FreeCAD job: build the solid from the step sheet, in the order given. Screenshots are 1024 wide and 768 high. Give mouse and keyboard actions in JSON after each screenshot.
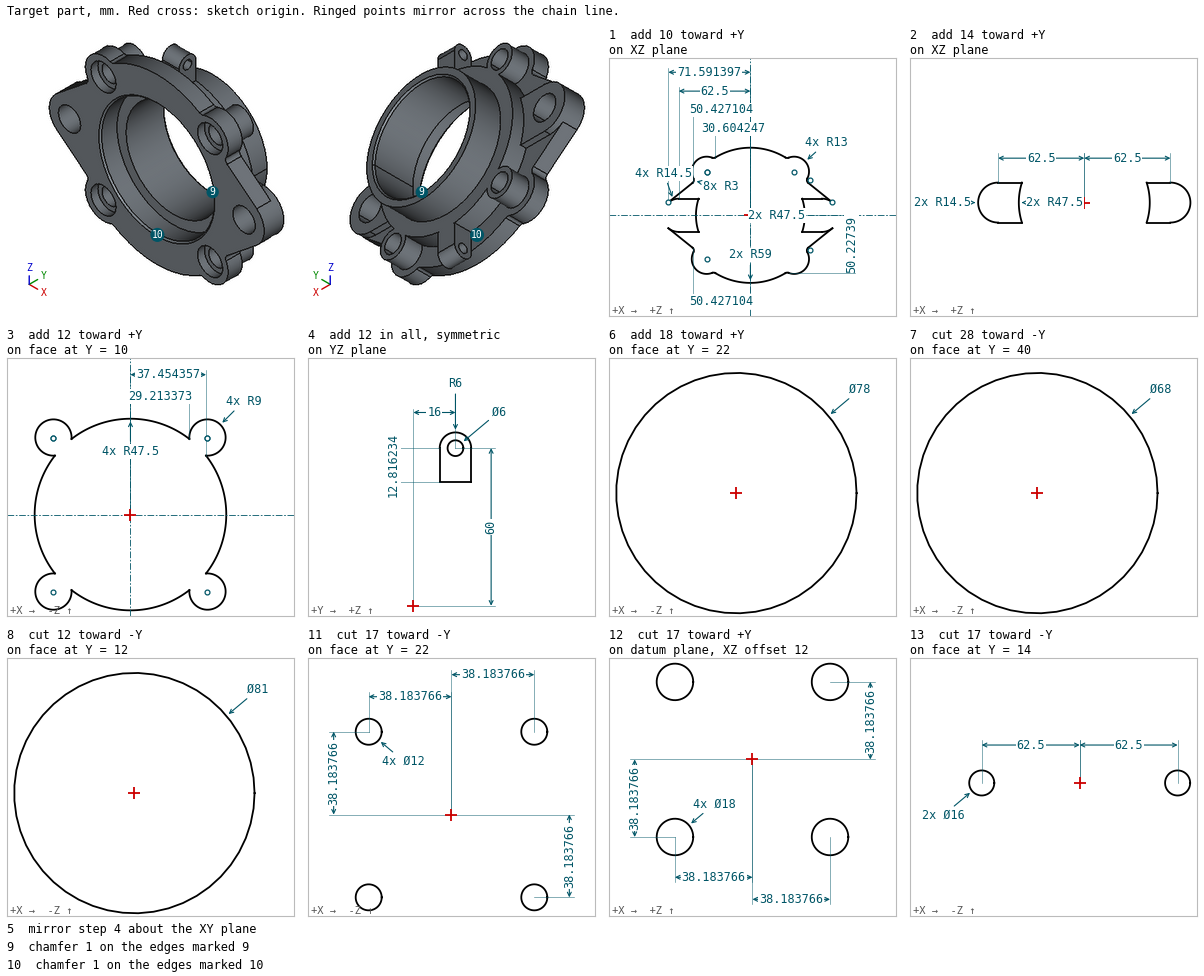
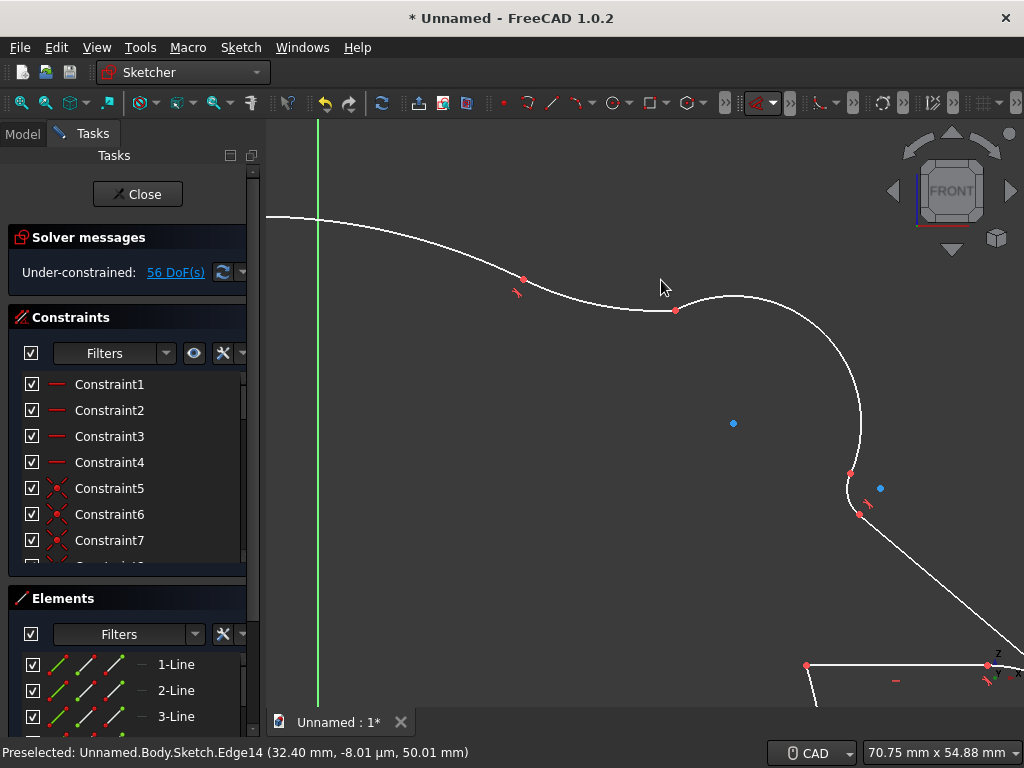
{"action": "scroll", "coordinate": [661, 281], "scroll_direction": "down", "scroll_amount": 7}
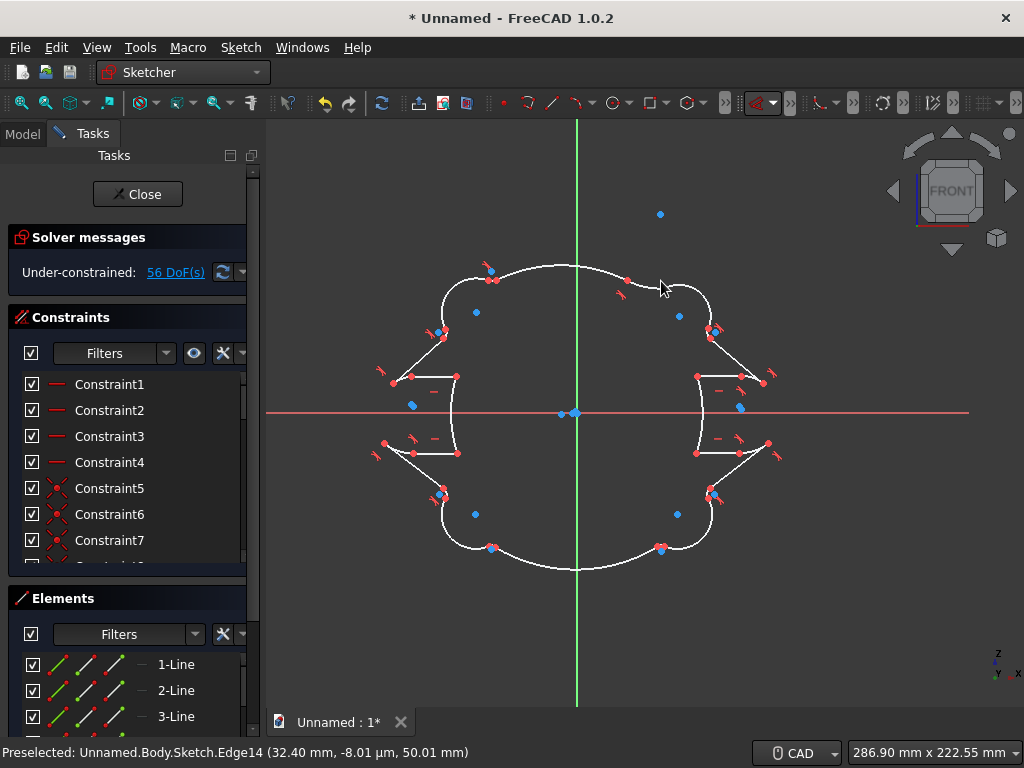
{"action": "left_click", "coordinate": [638, 285]}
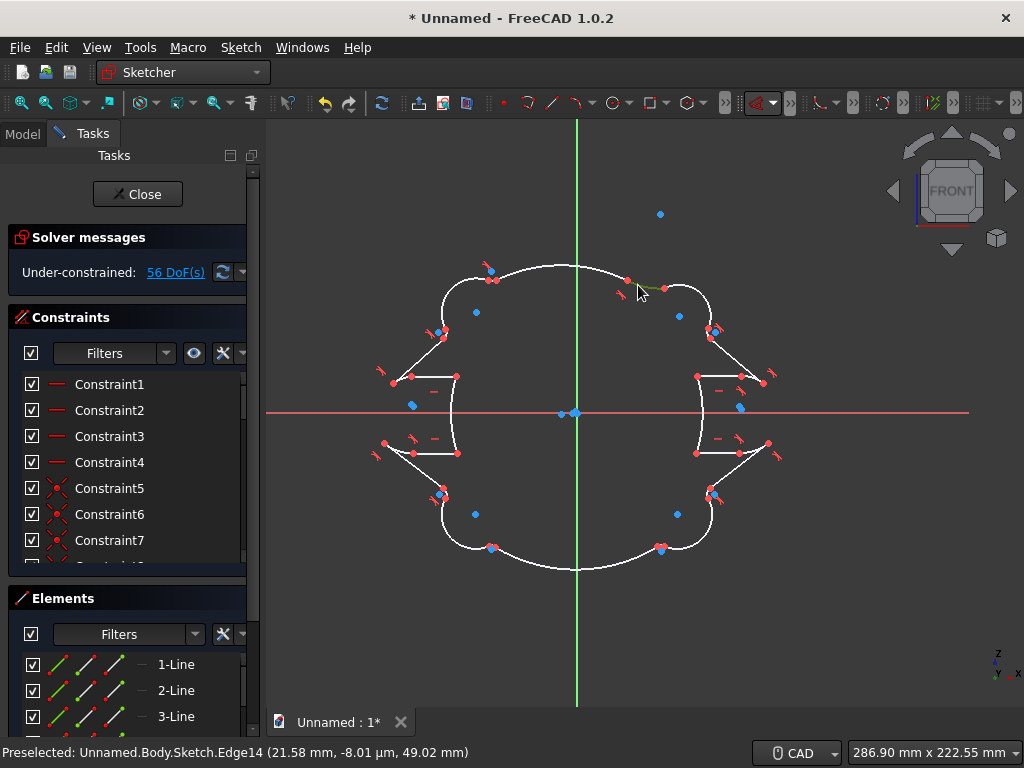
{"action": "left_click", "coordinate": [709, 306]}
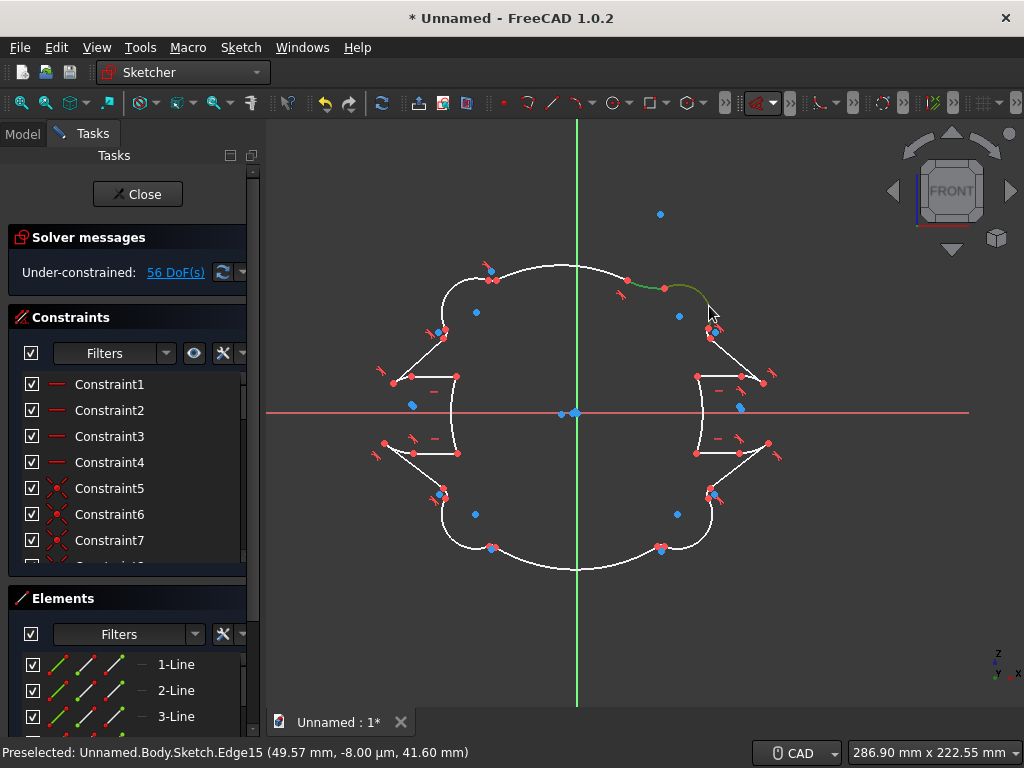
{"action": "key", "text": "t"}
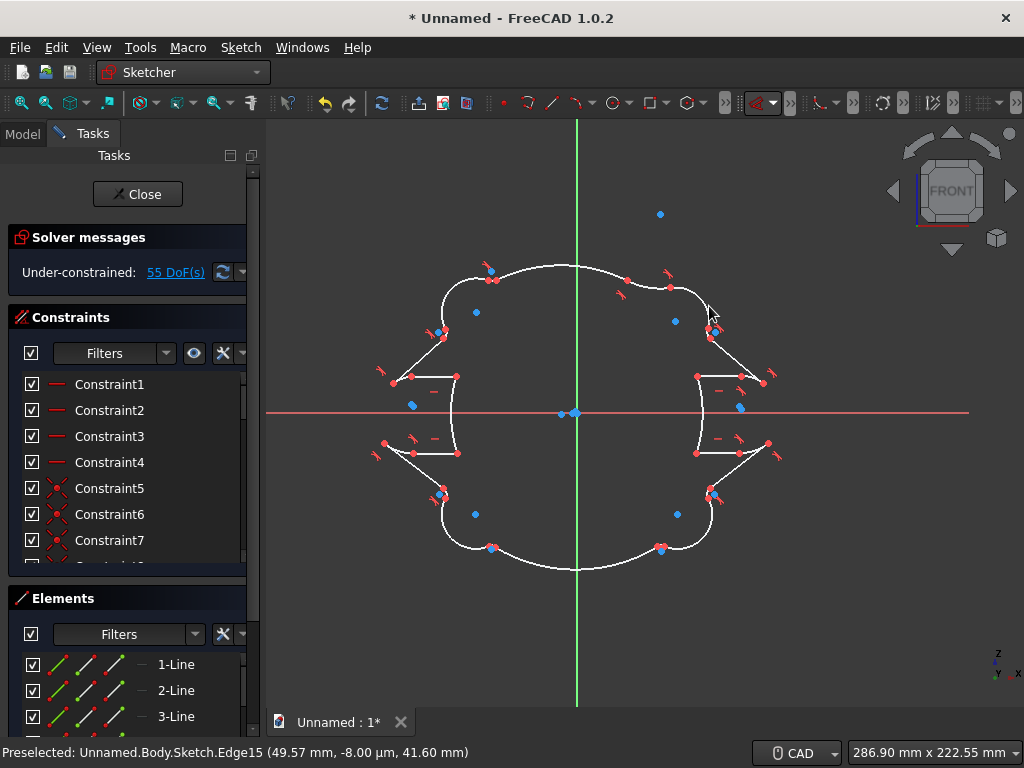
{"action": "left_click", "coordinate": [707, 309]}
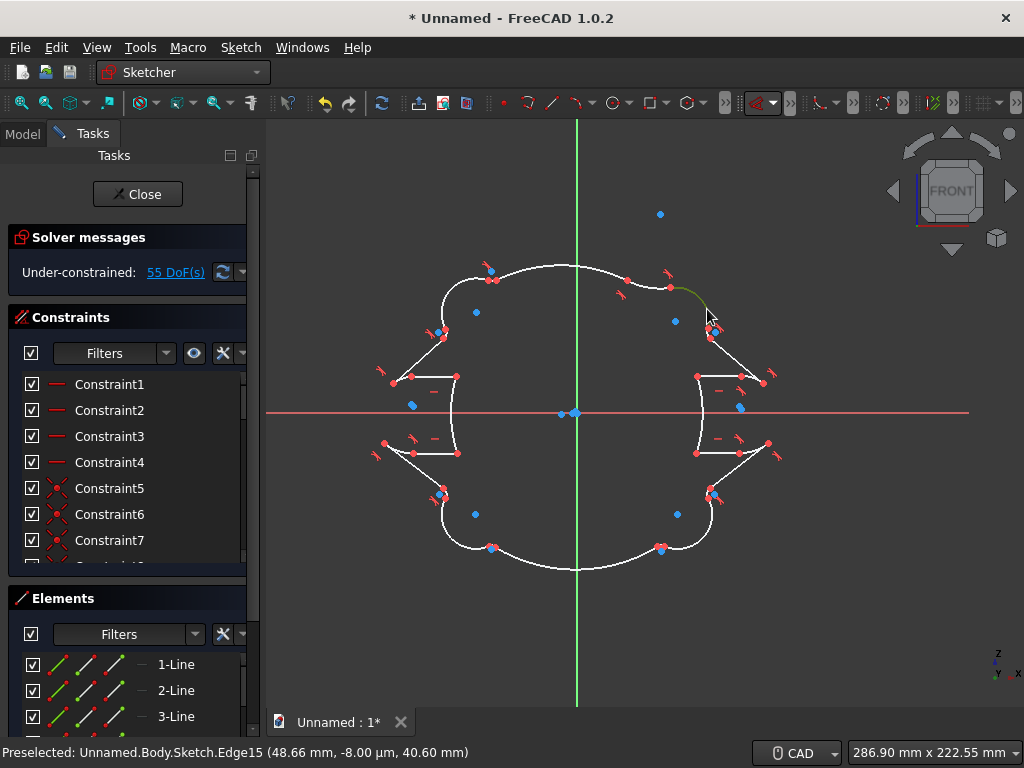
{"action": "scroll", "coordinate": [707, 334], "scroll_direction": "up", "scroll_amount": 5}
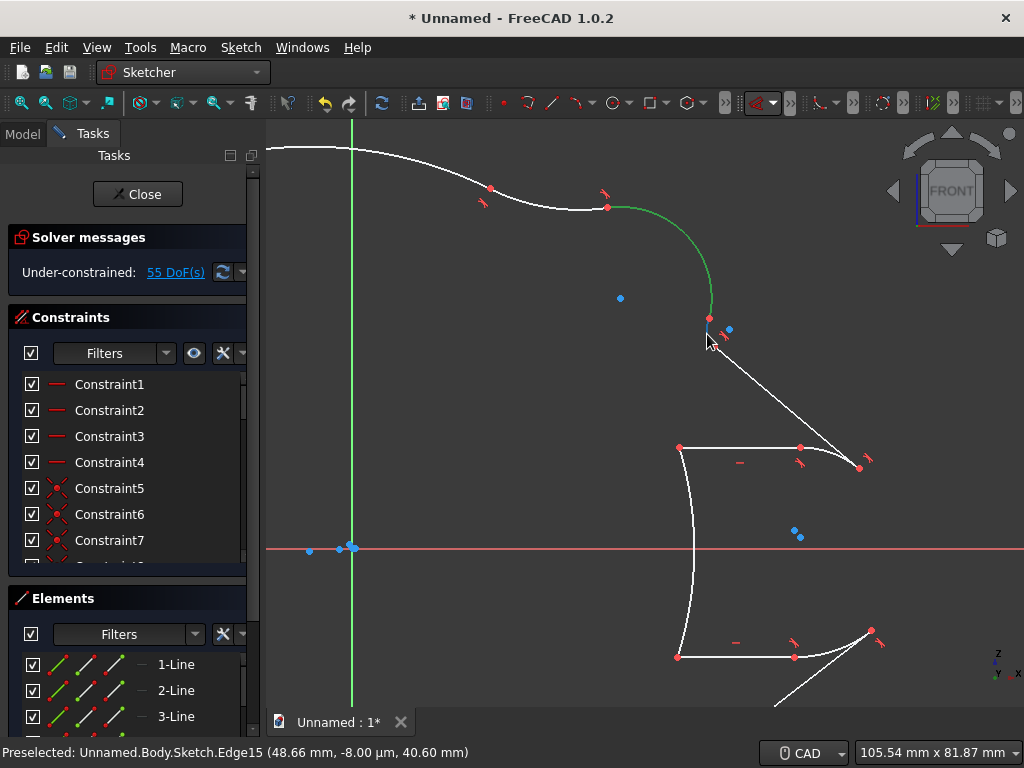
{"action": "left_click", "coordinate": [707, 334]}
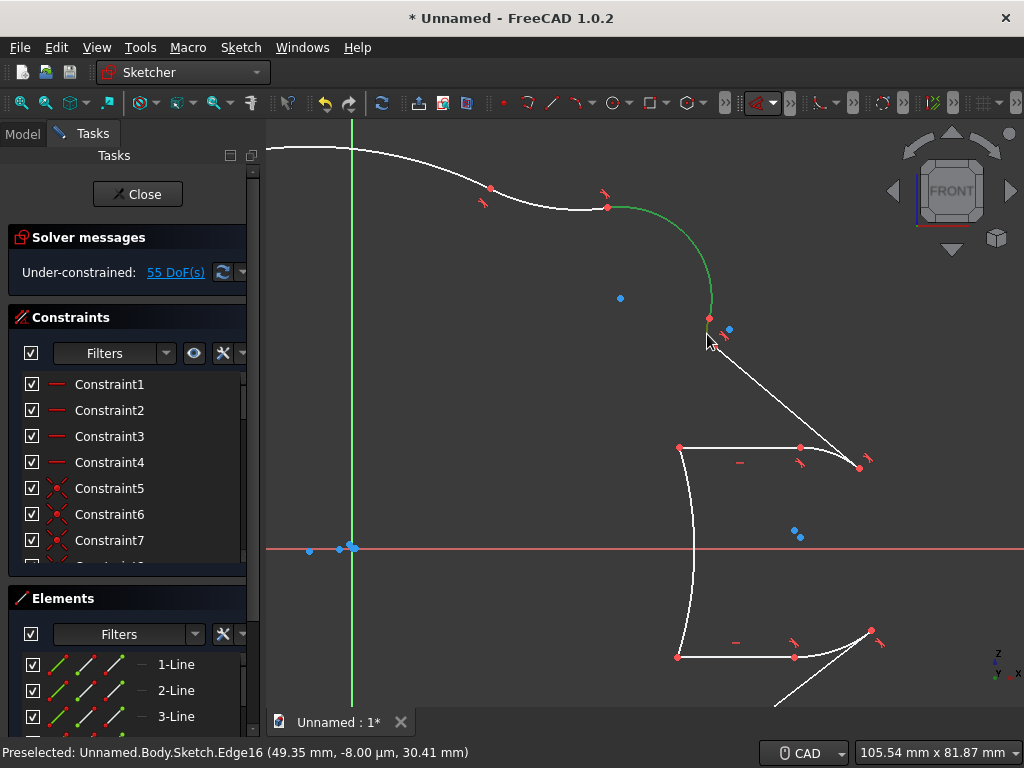
{"action": "key", "text": "t"}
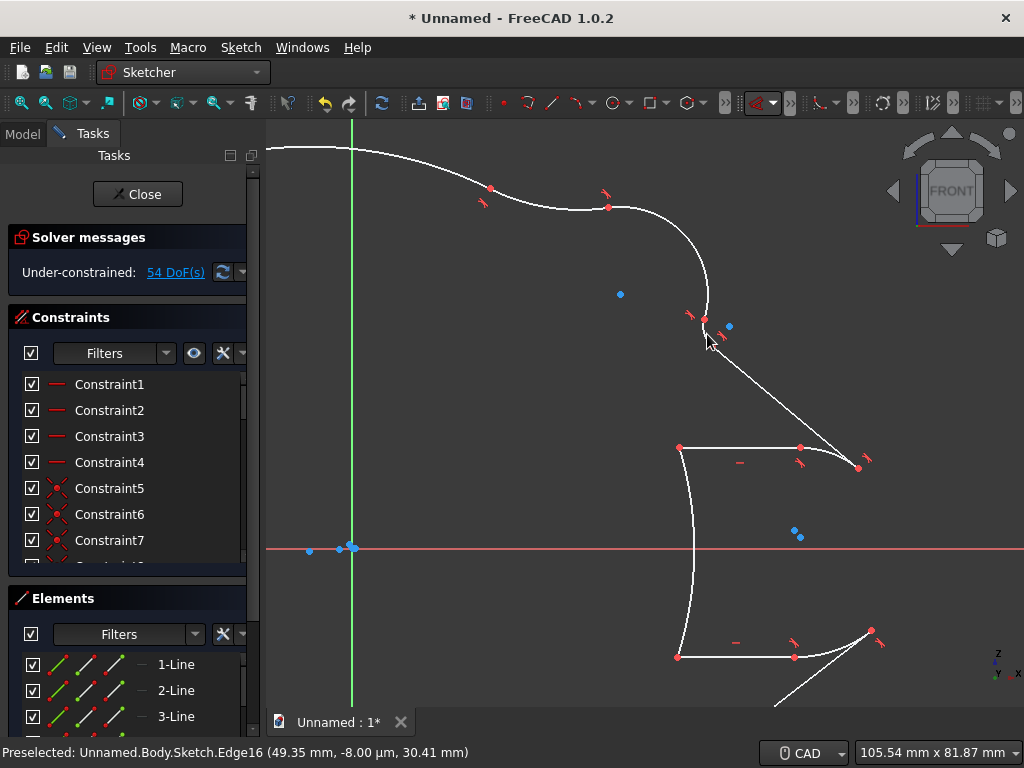
{"action": "scroll", "coordinate": [707, 334], "scroll_direction": "down", "scroll_amount": 5}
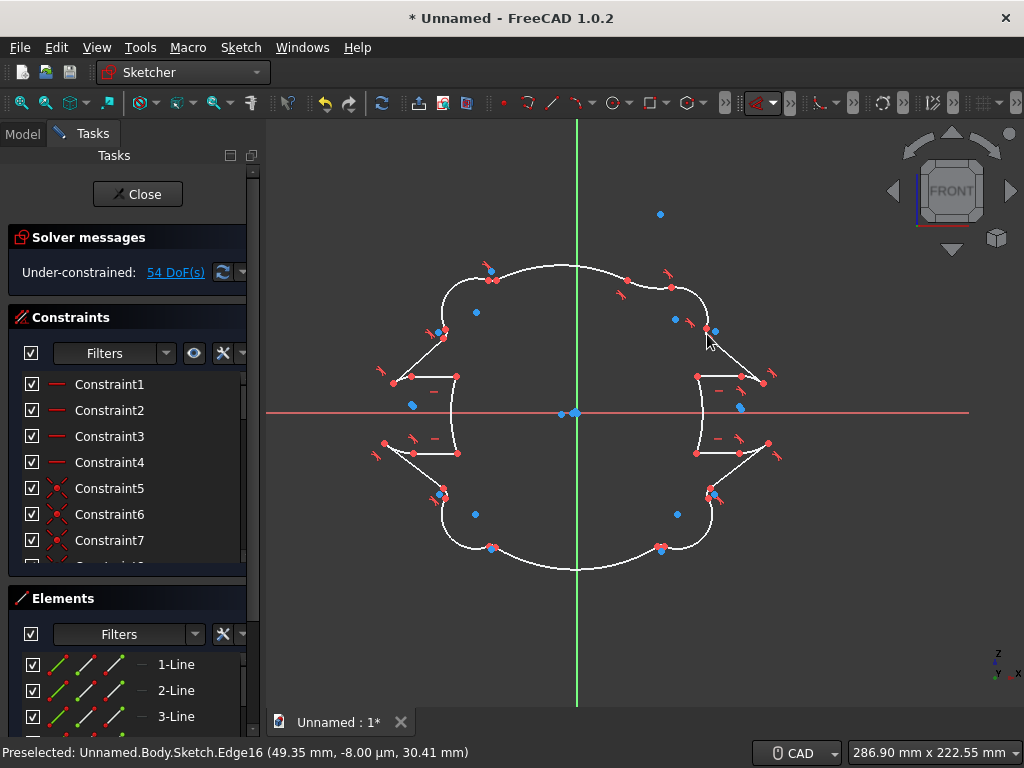
{"action": "scroll", "coordinate": [707, 493], "scroll_direction": "up", "scroll_amount": 5}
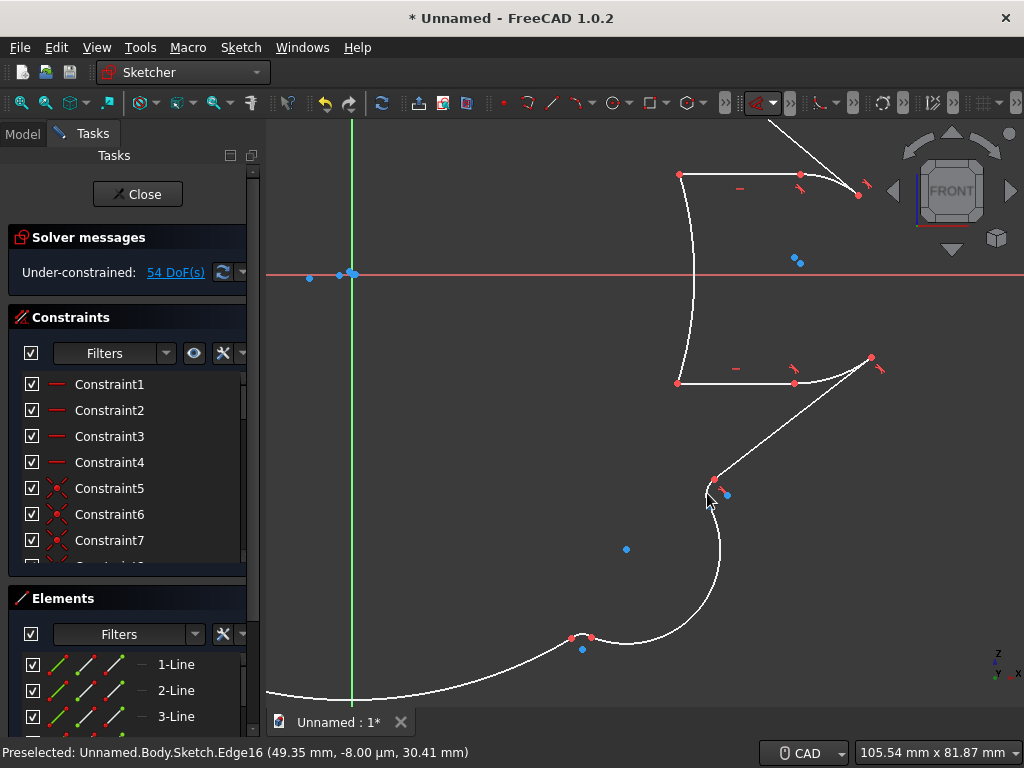
{"action": "left_click", "coordinate": [707, 492]}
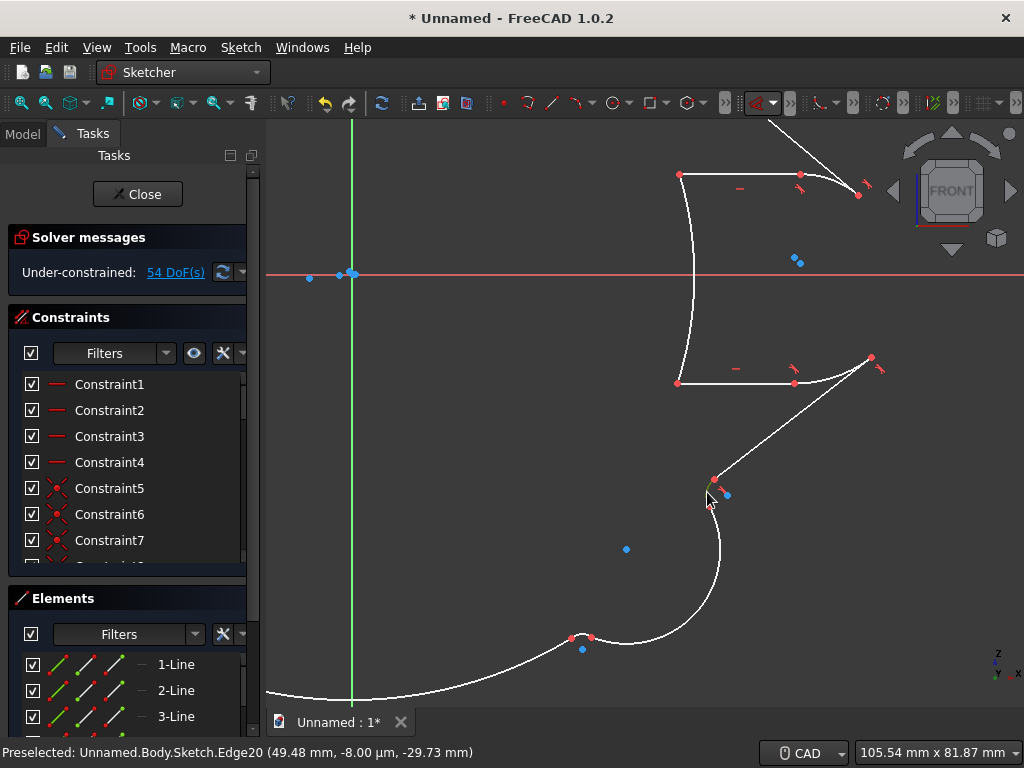
{"action": "left_click", "coordinate": [658, 638]}